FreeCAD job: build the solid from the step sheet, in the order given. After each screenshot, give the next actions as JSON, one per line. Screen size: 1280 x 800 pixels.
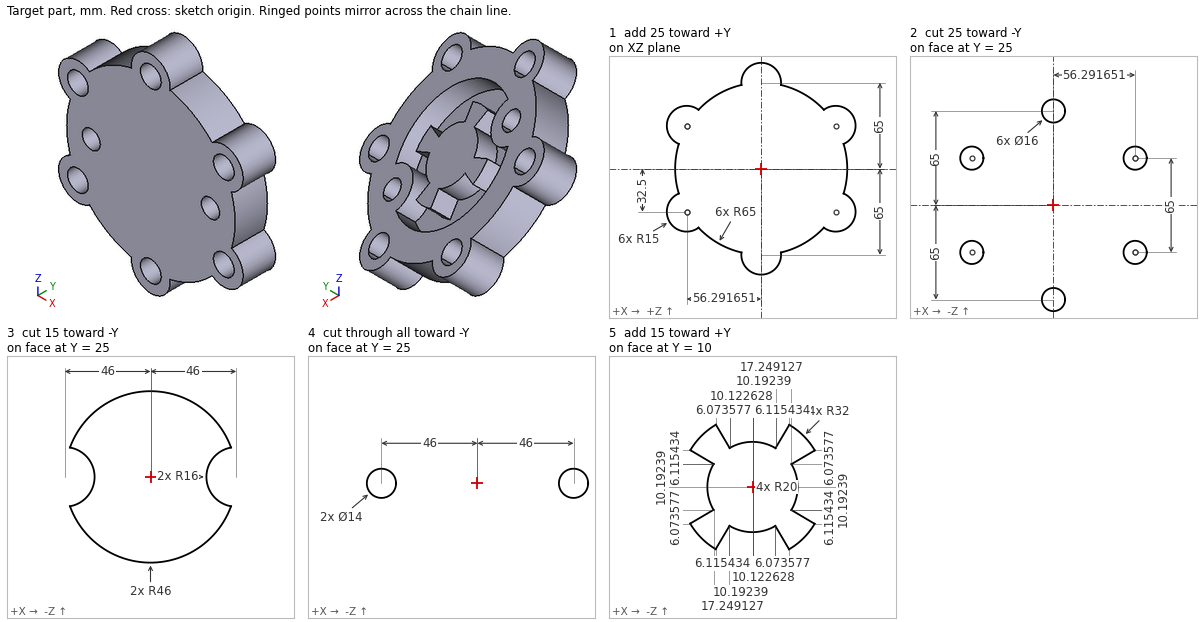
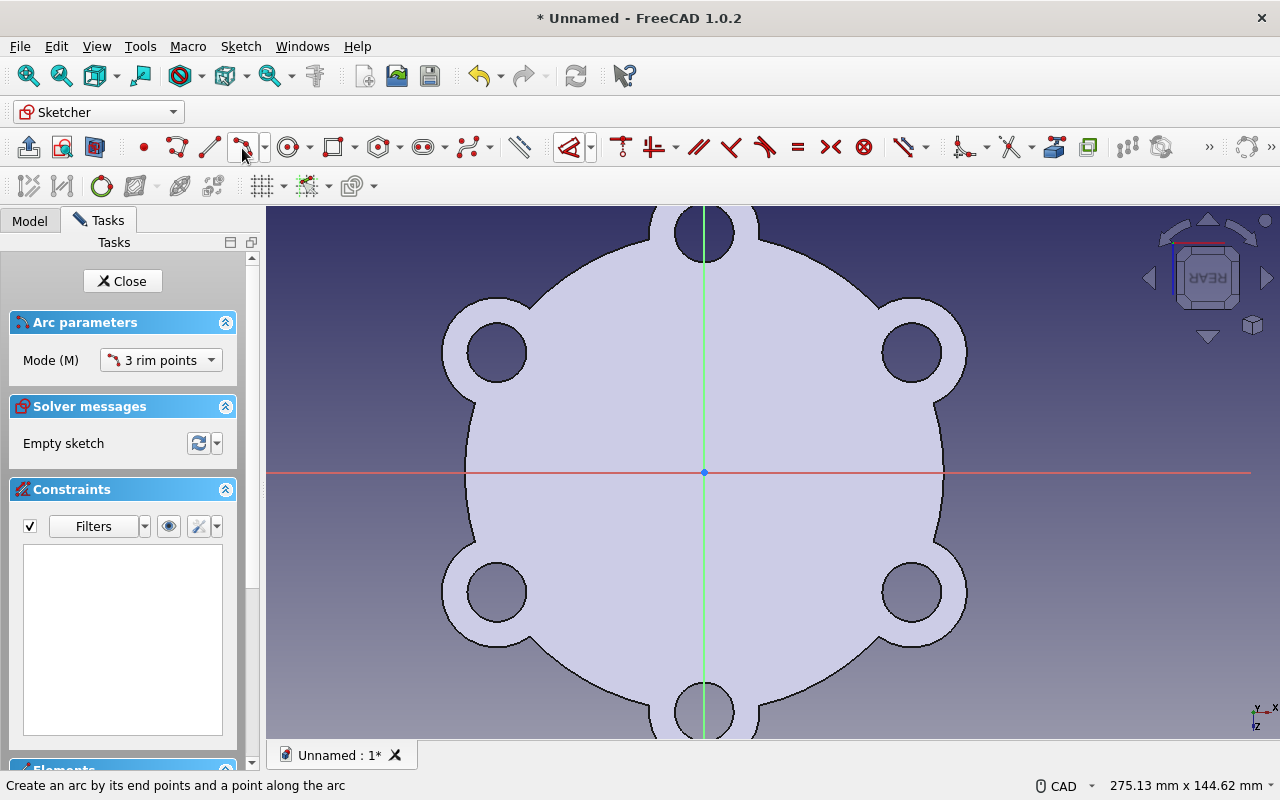
{"action": "left_click", "coordinate": [545, 531]}
{"action": "left_click", "coordinate": [864, 531]}
{"action": "left_click", "coordinate": [663, 637]}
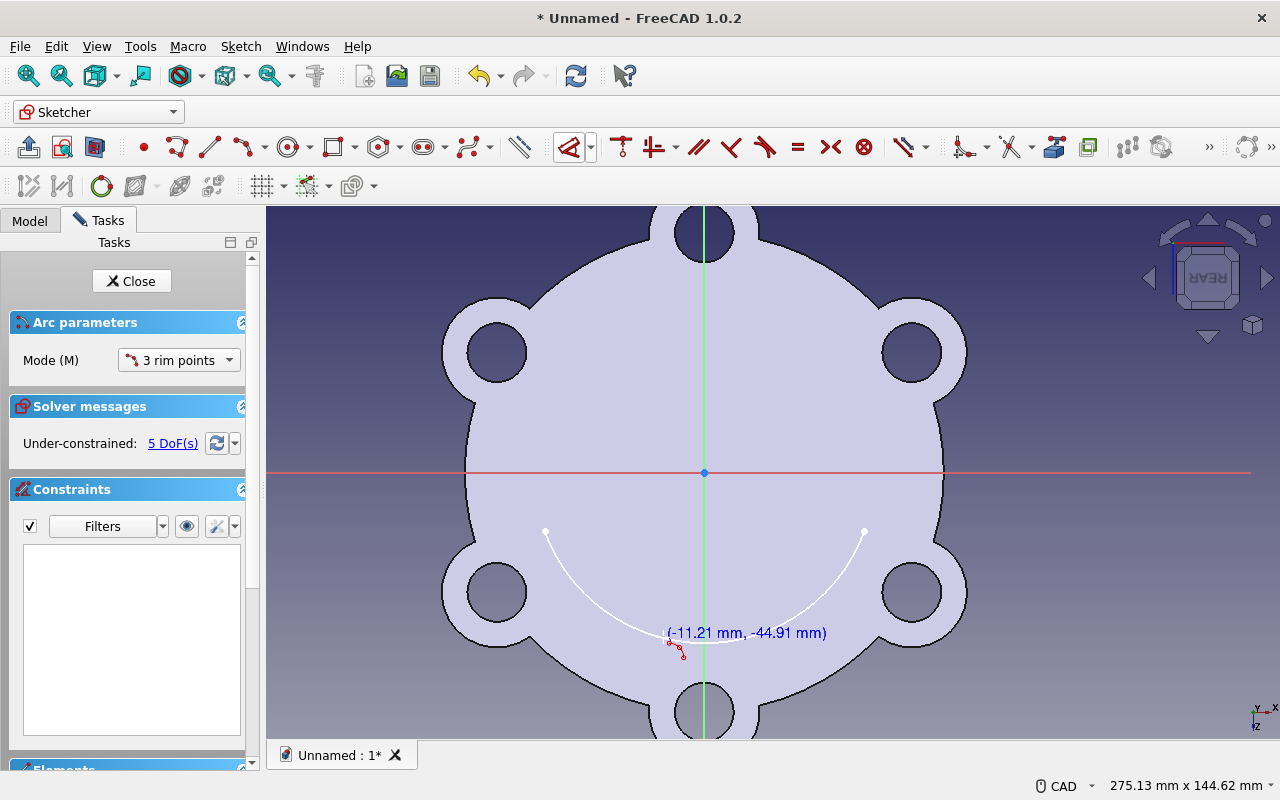
{"action": "left_click", "coordinate": [864, 532]}
{"action": "left_click", "coordinate": [864, 414]}
{"action": "left_click", "coordinate": [817, 456]}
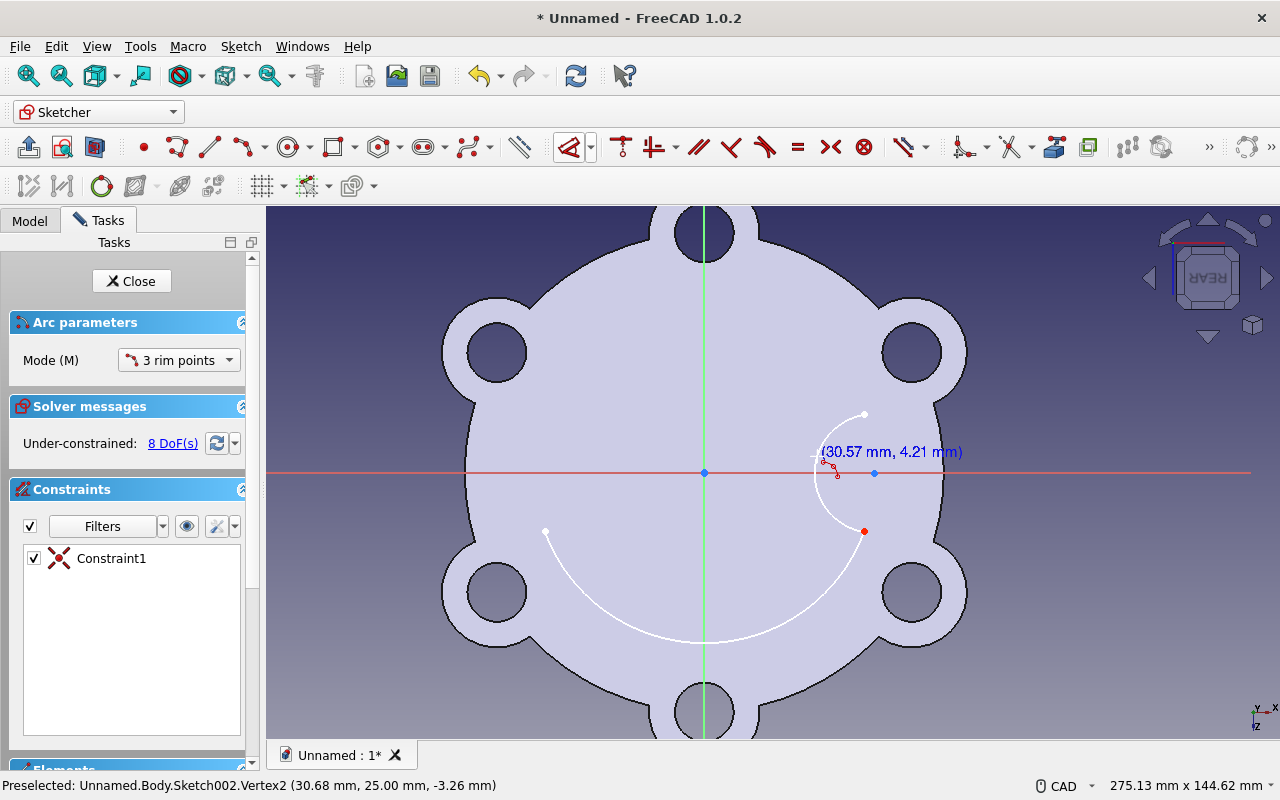
{"action": "left_click", "coordinate": [864, 415]}
{"action": "left_click", "coordinate": [545, 414]}
{"action": "left_click", "coordinate": [745, 308]}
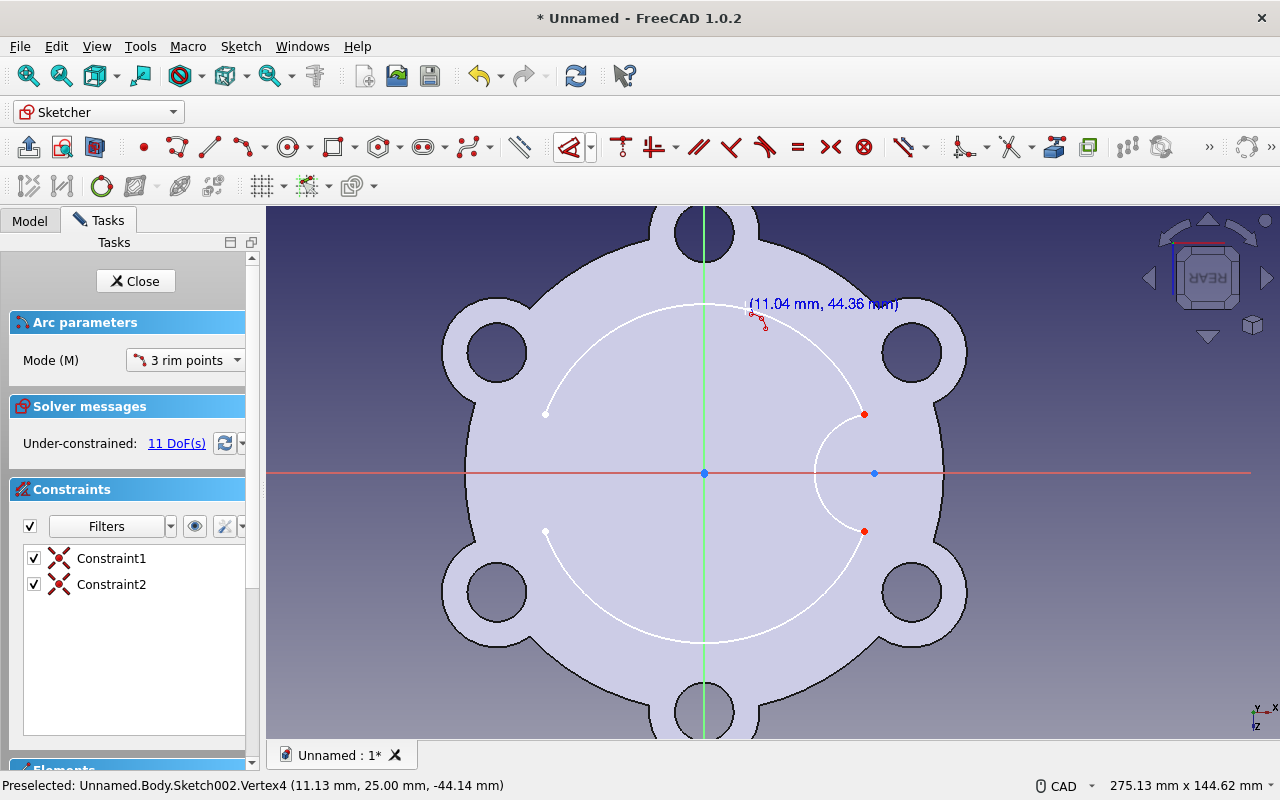
{"action": "left_click", "coordinate": [545, 415]}
{"action": "left_click", "coordinate": [545, 532]}
{"action": "left_click", "coordinate": [591, 489]}
{"action": "key", "text": "Escape"}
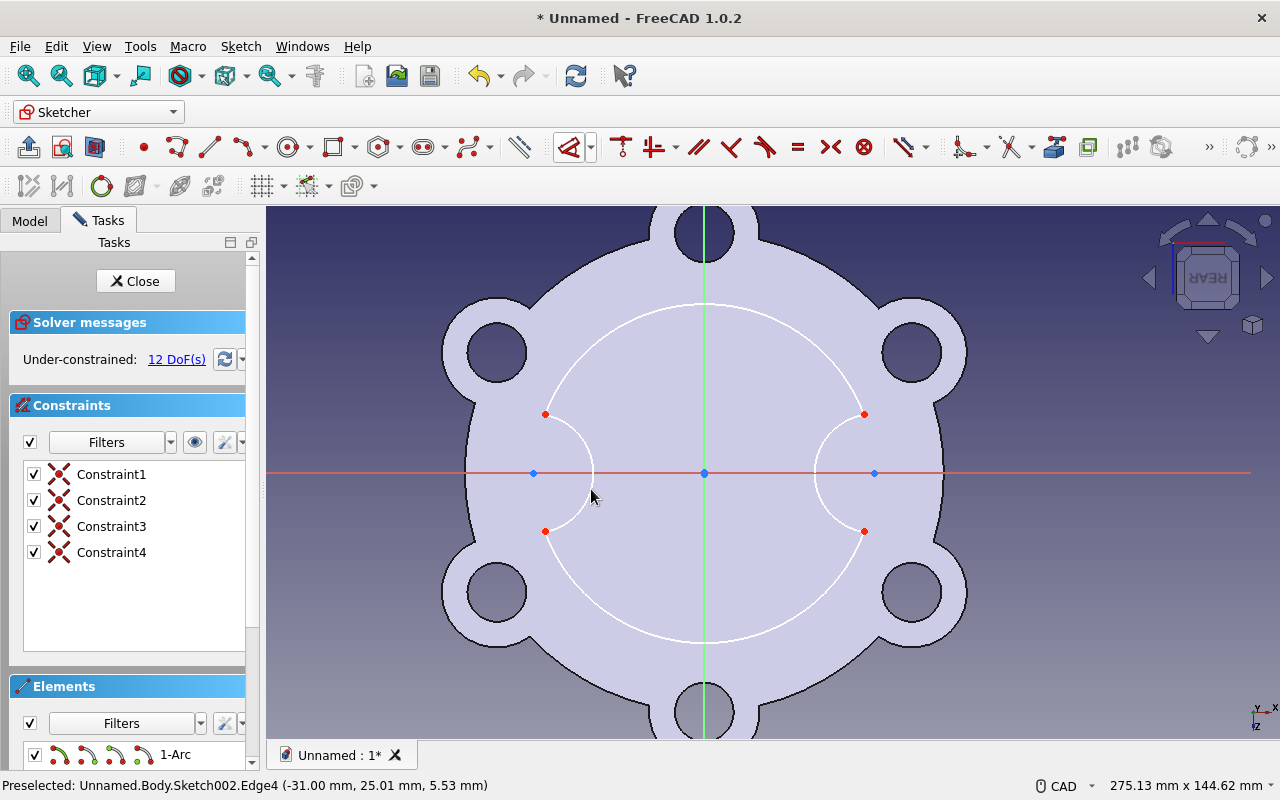
{"action": "left_click", "coordinate": [625, 623]}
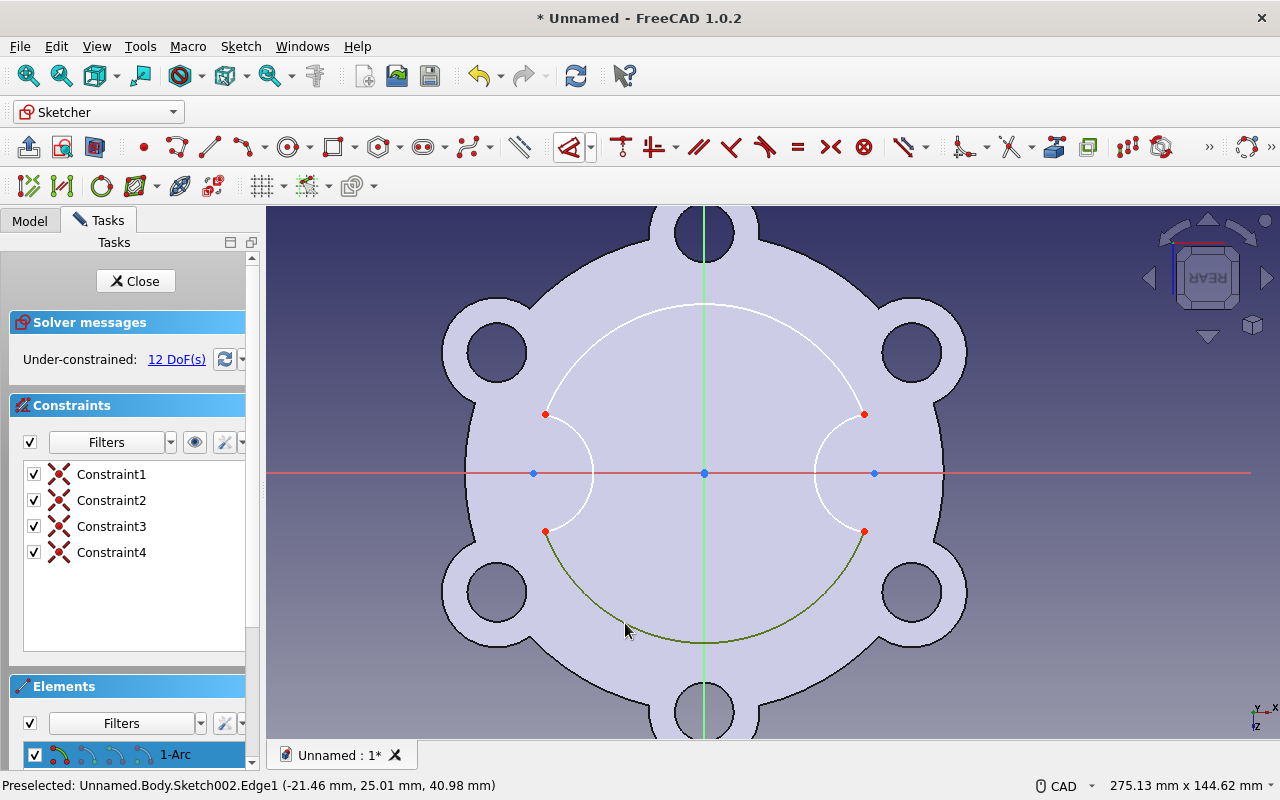
{"action": "left_click", "coordinate": [784, 324]}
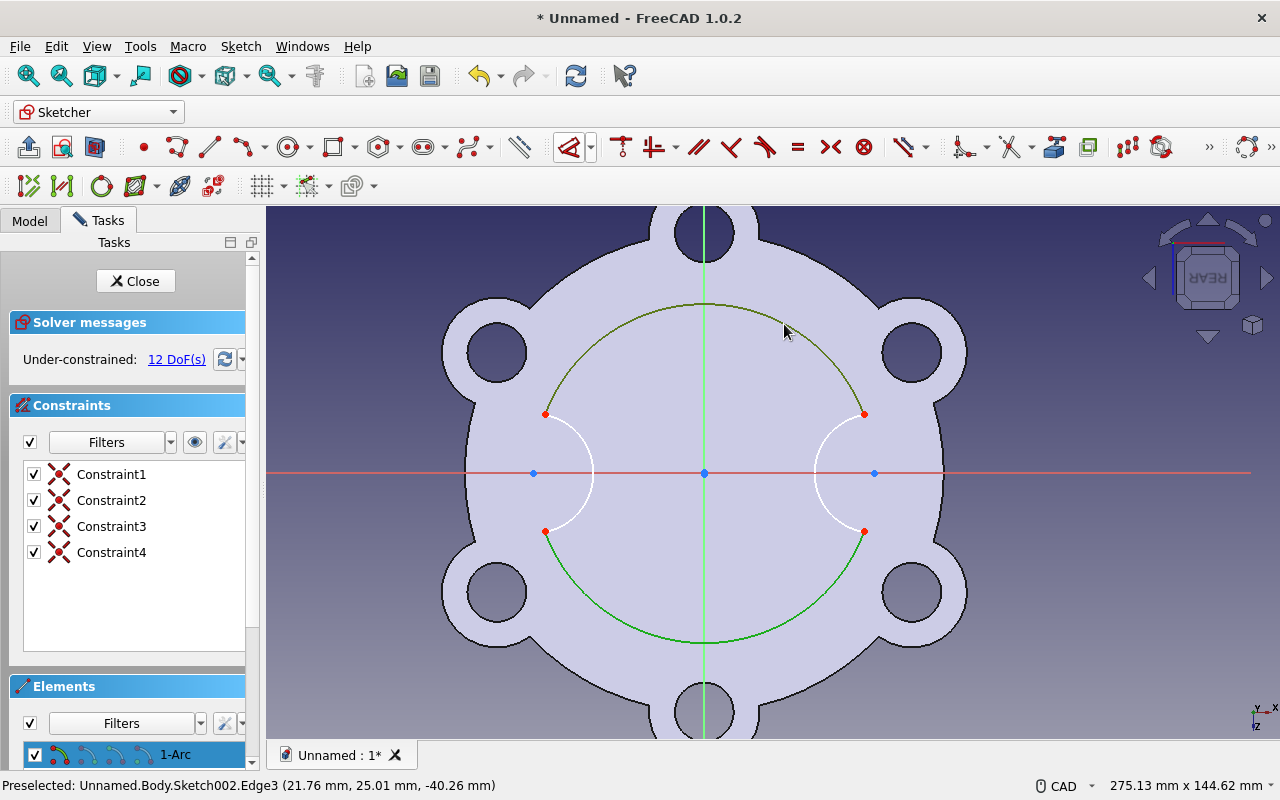
{"action": "left_click", "coordinate": [621, 148]}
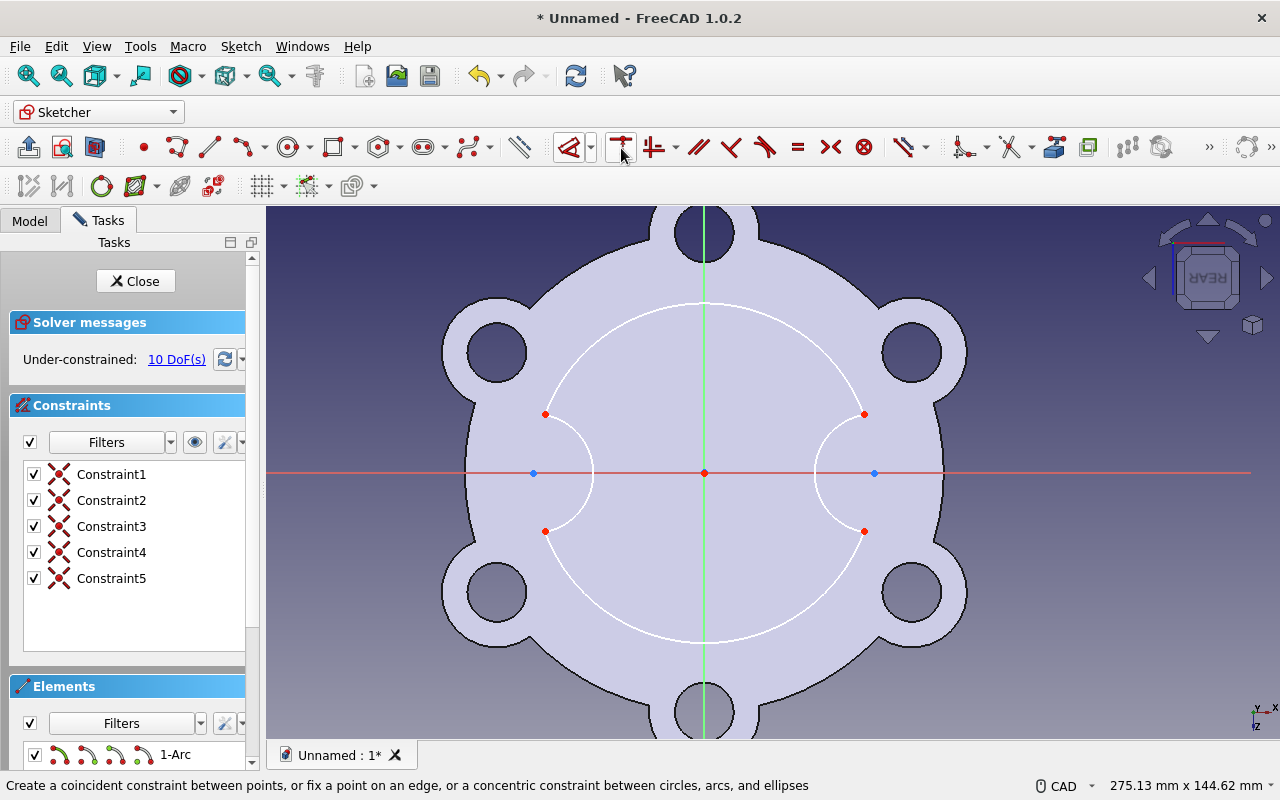
{"action": "left_click_drag", "start_coordinate": [694, 462], "coordinate": [715, 483]}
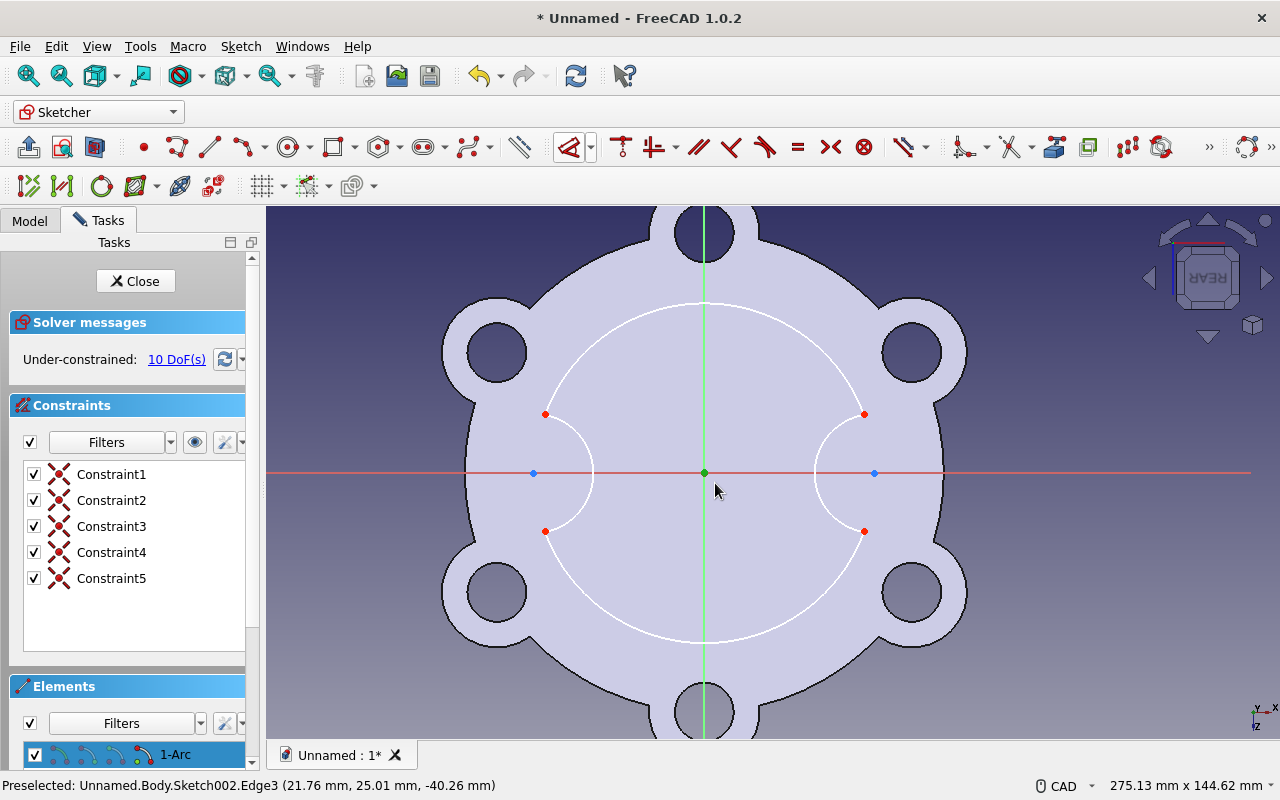
{"action": "left_click", "coordinate": [621, 148]}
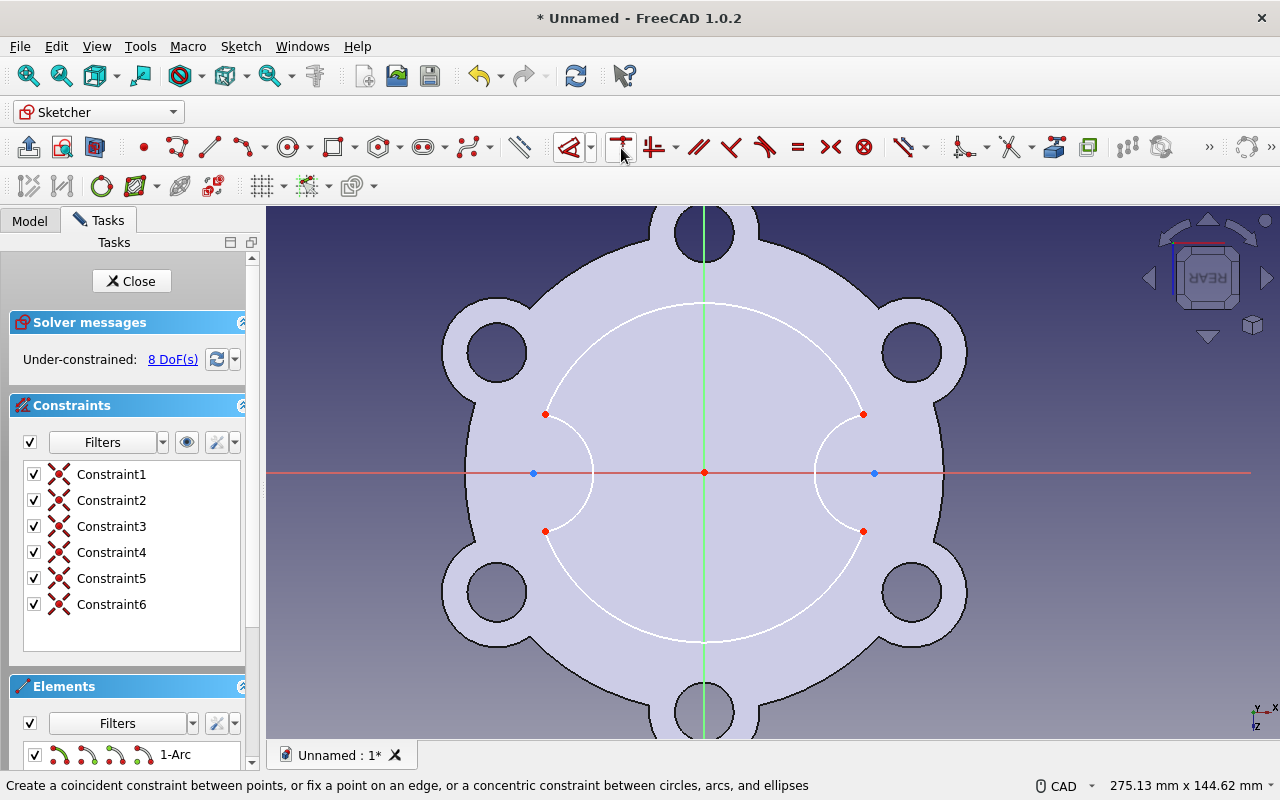
{"action": "left_click", "coordinate": [625, 623]}